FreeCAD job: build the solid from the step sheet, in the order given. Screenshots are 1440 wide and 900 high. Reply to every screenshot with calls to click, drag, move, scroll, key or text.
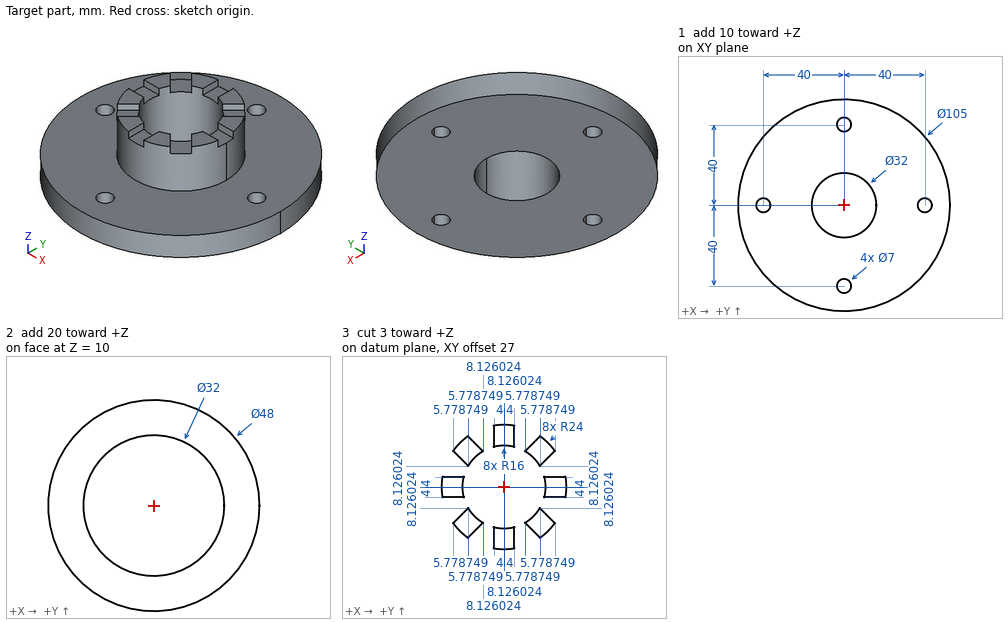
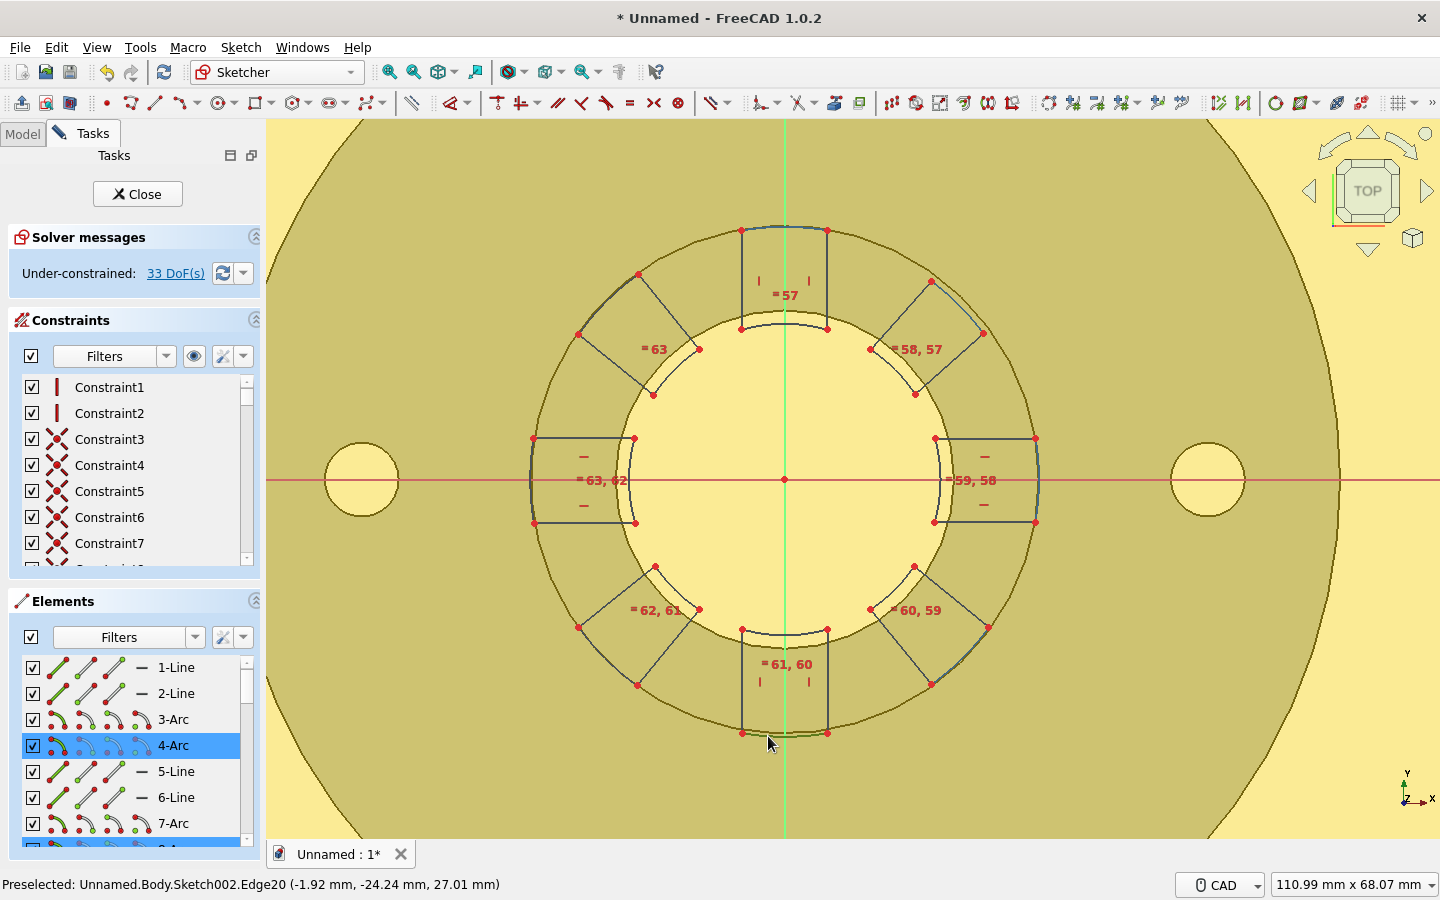
click(594, 647)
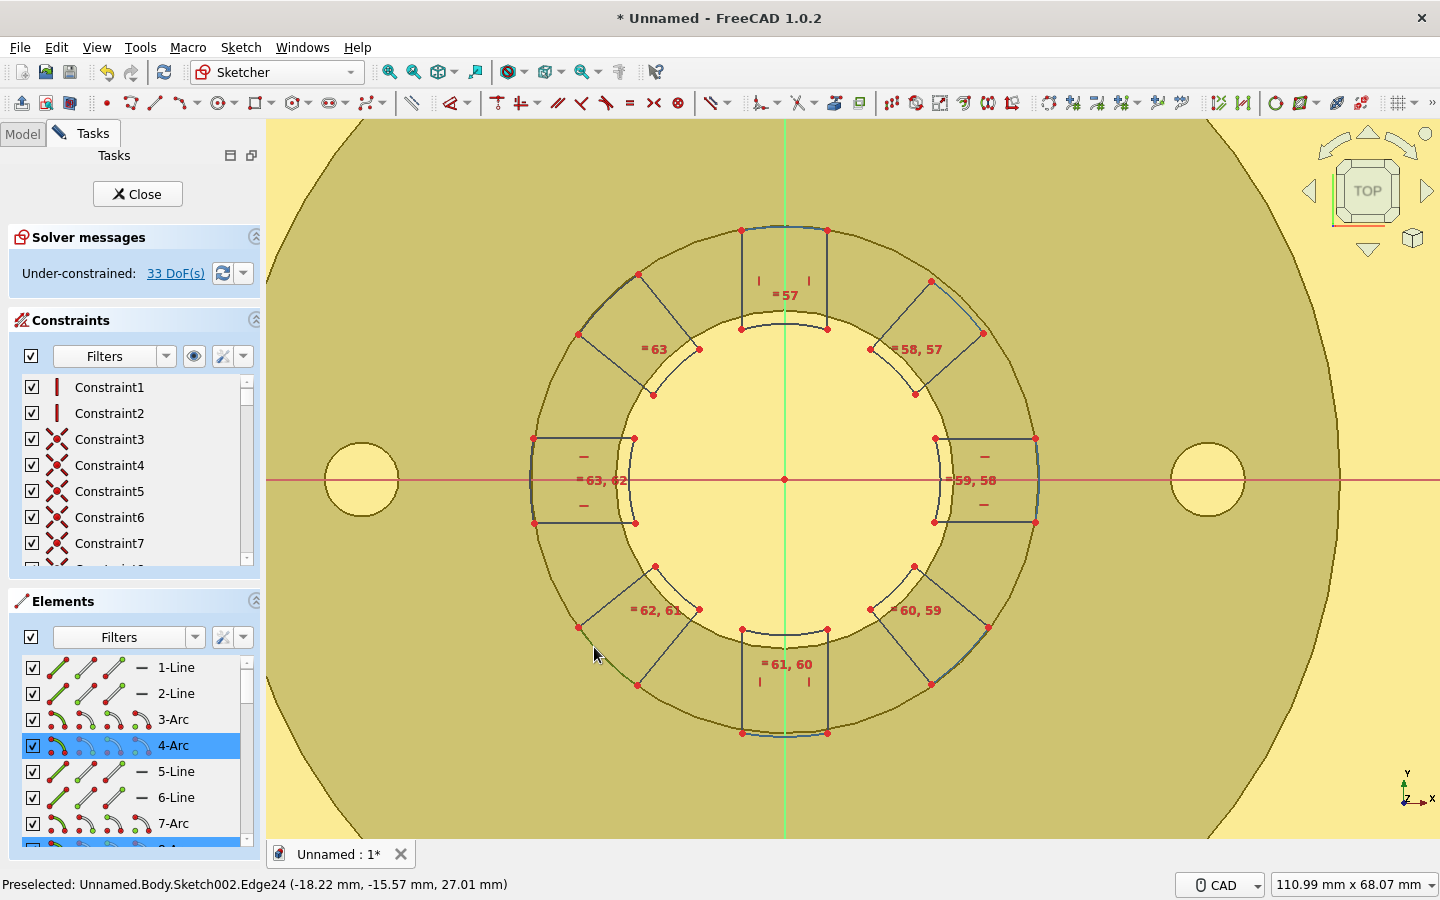
click(531, 464)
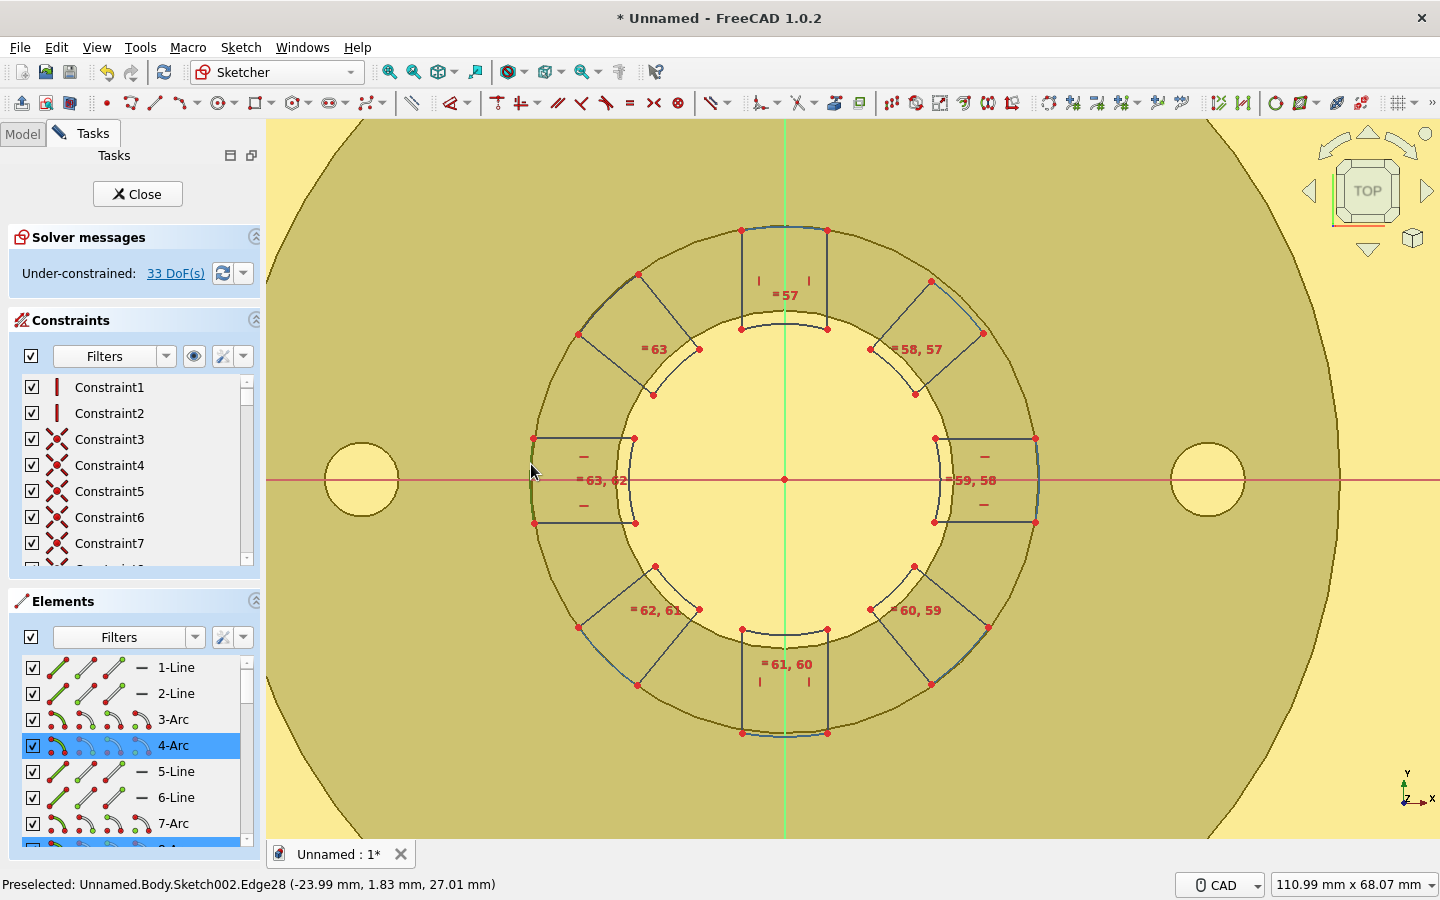
click(618, 290)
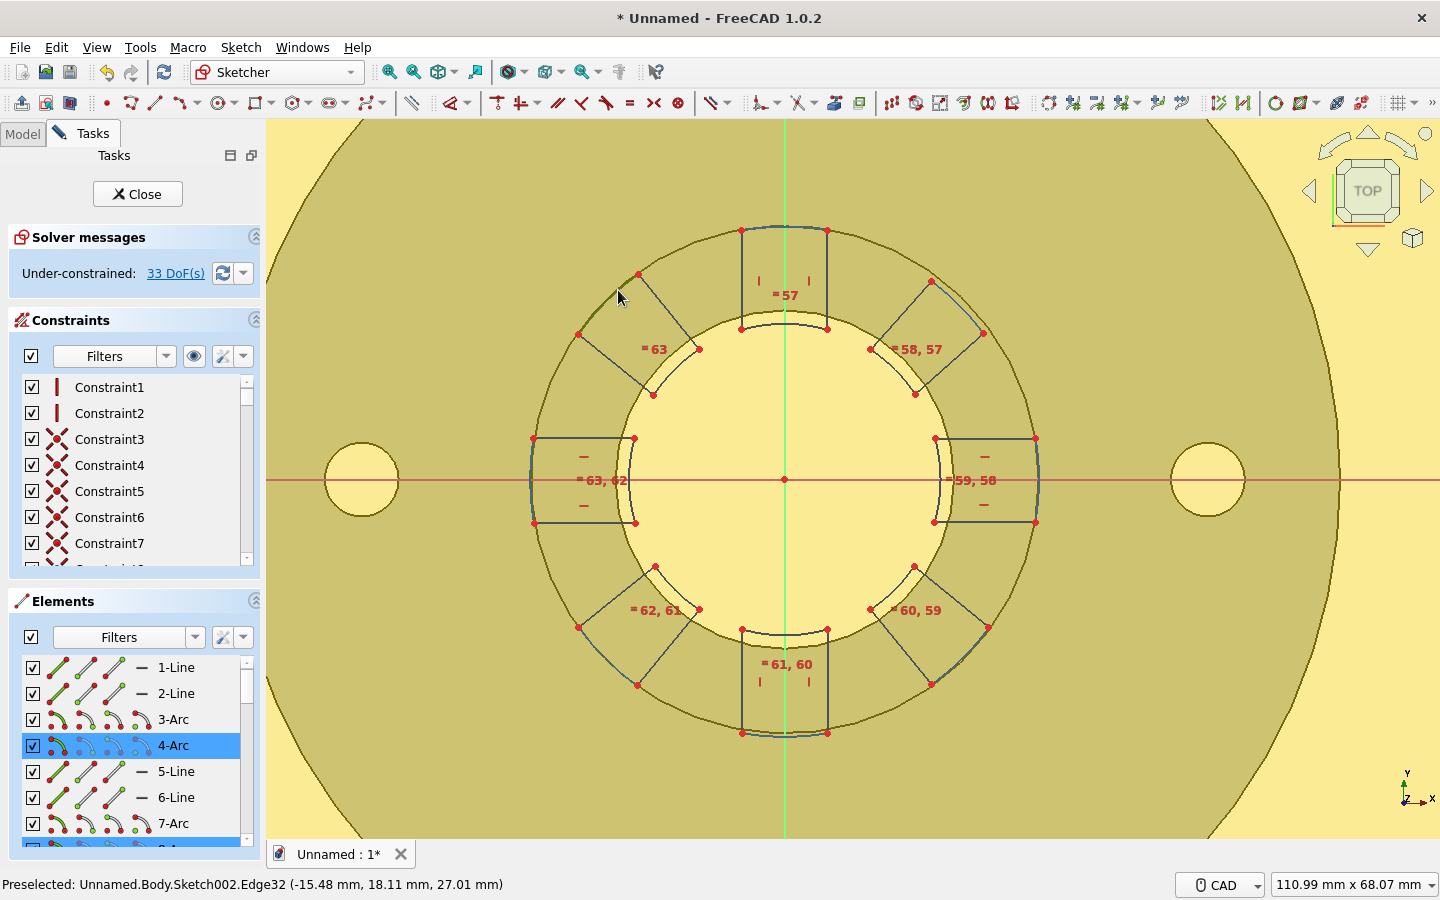
click(630, 104)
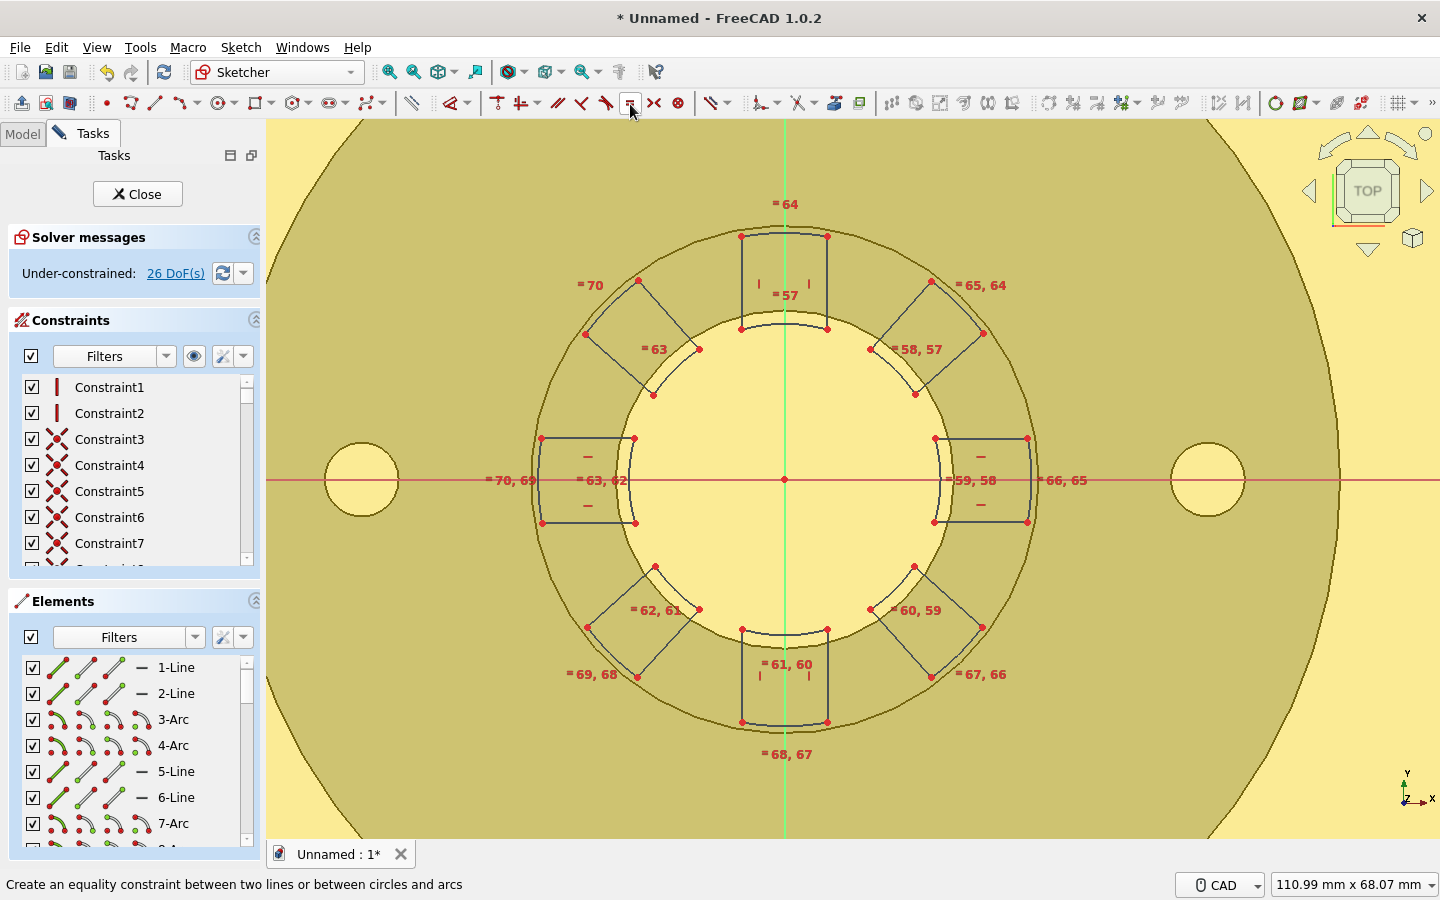
click(450, 104)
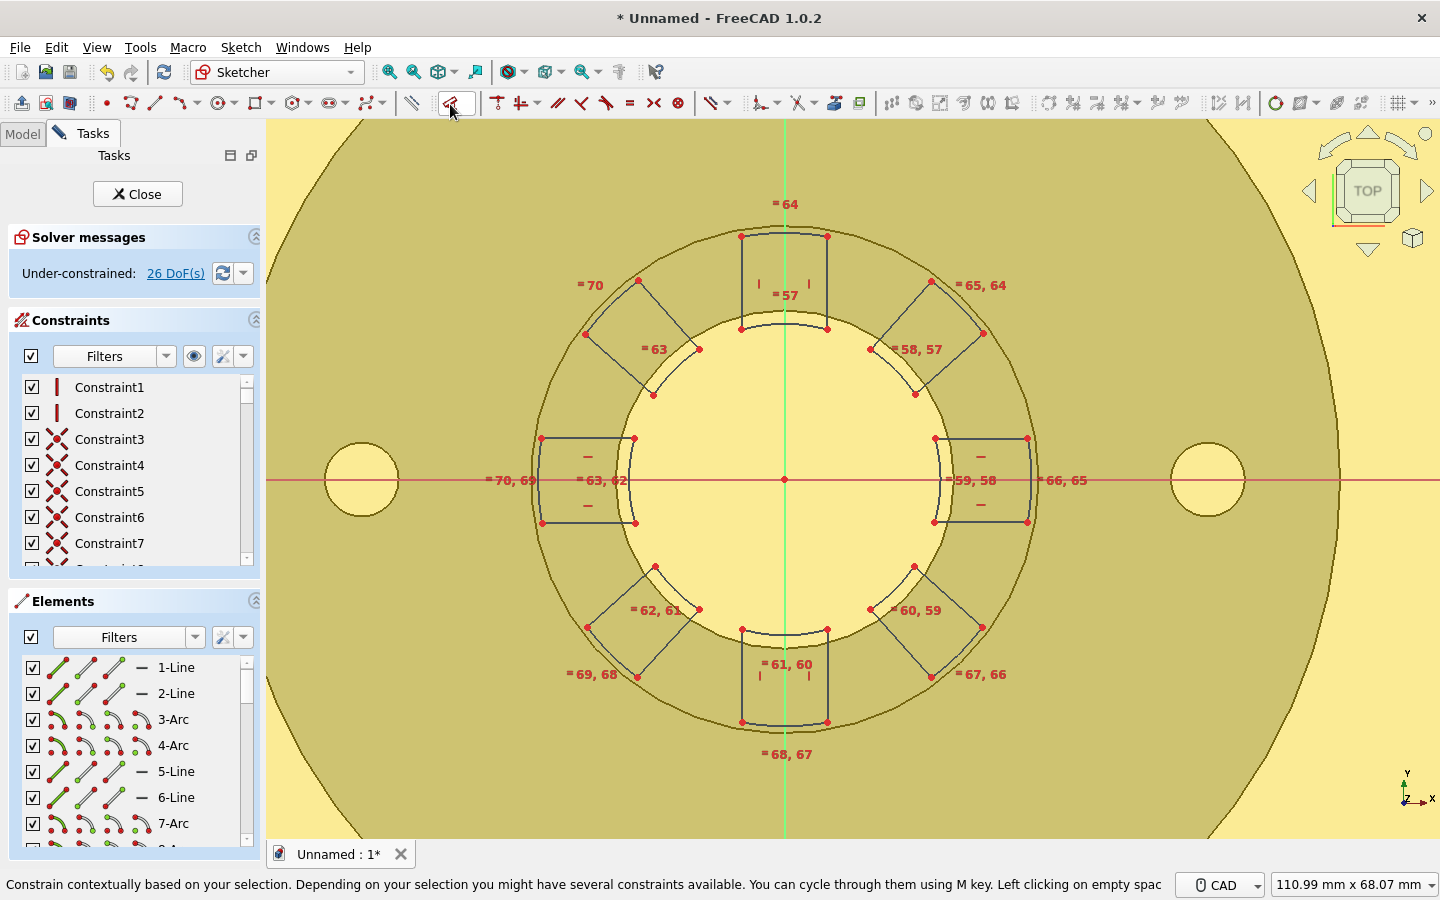
click(802, 325)
click(806, 293)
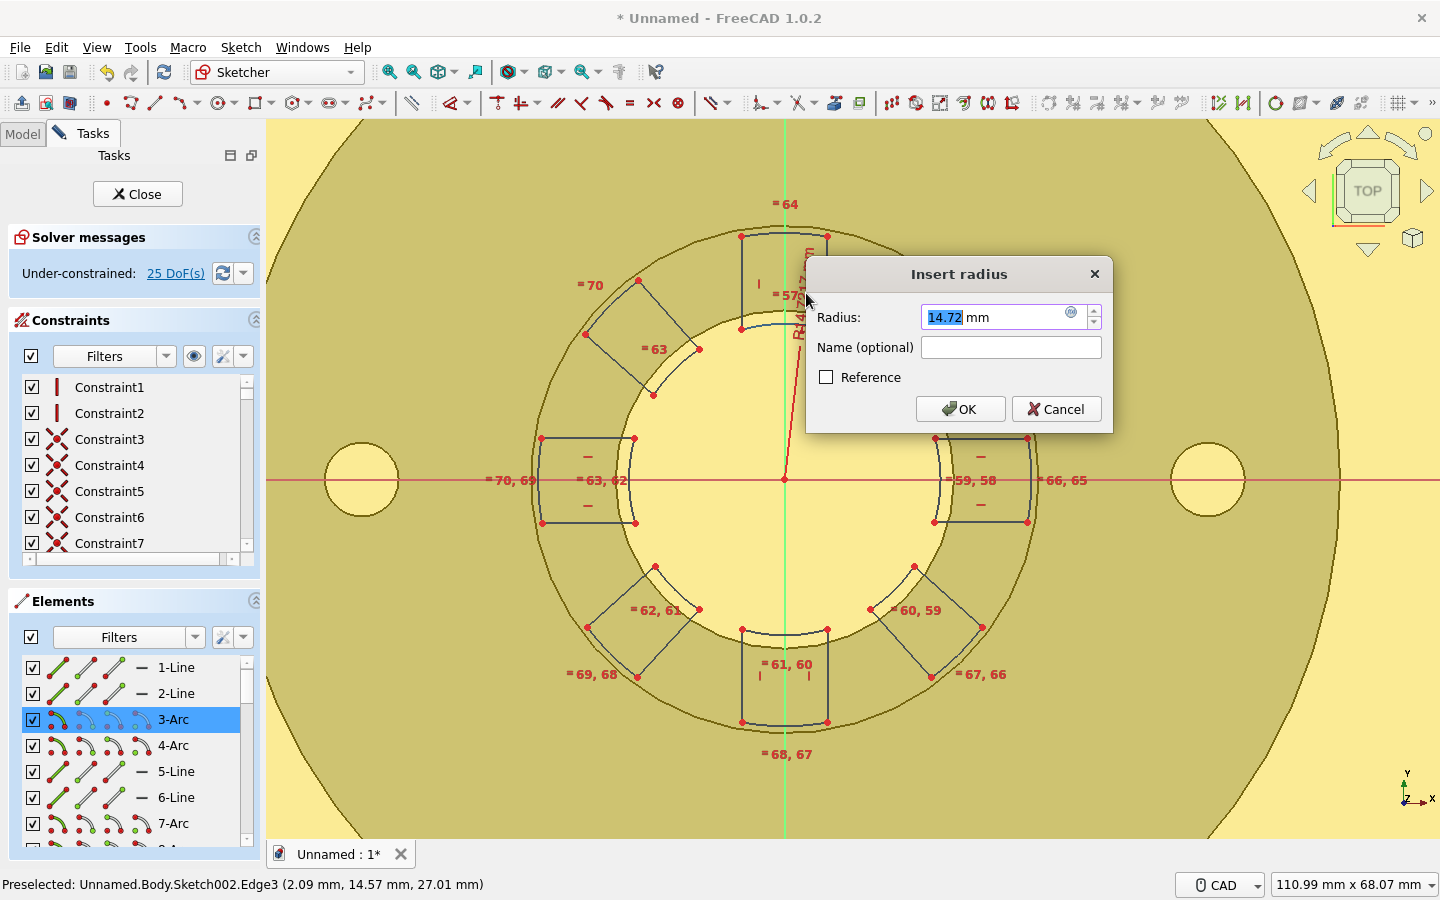
text(16)
key(Return)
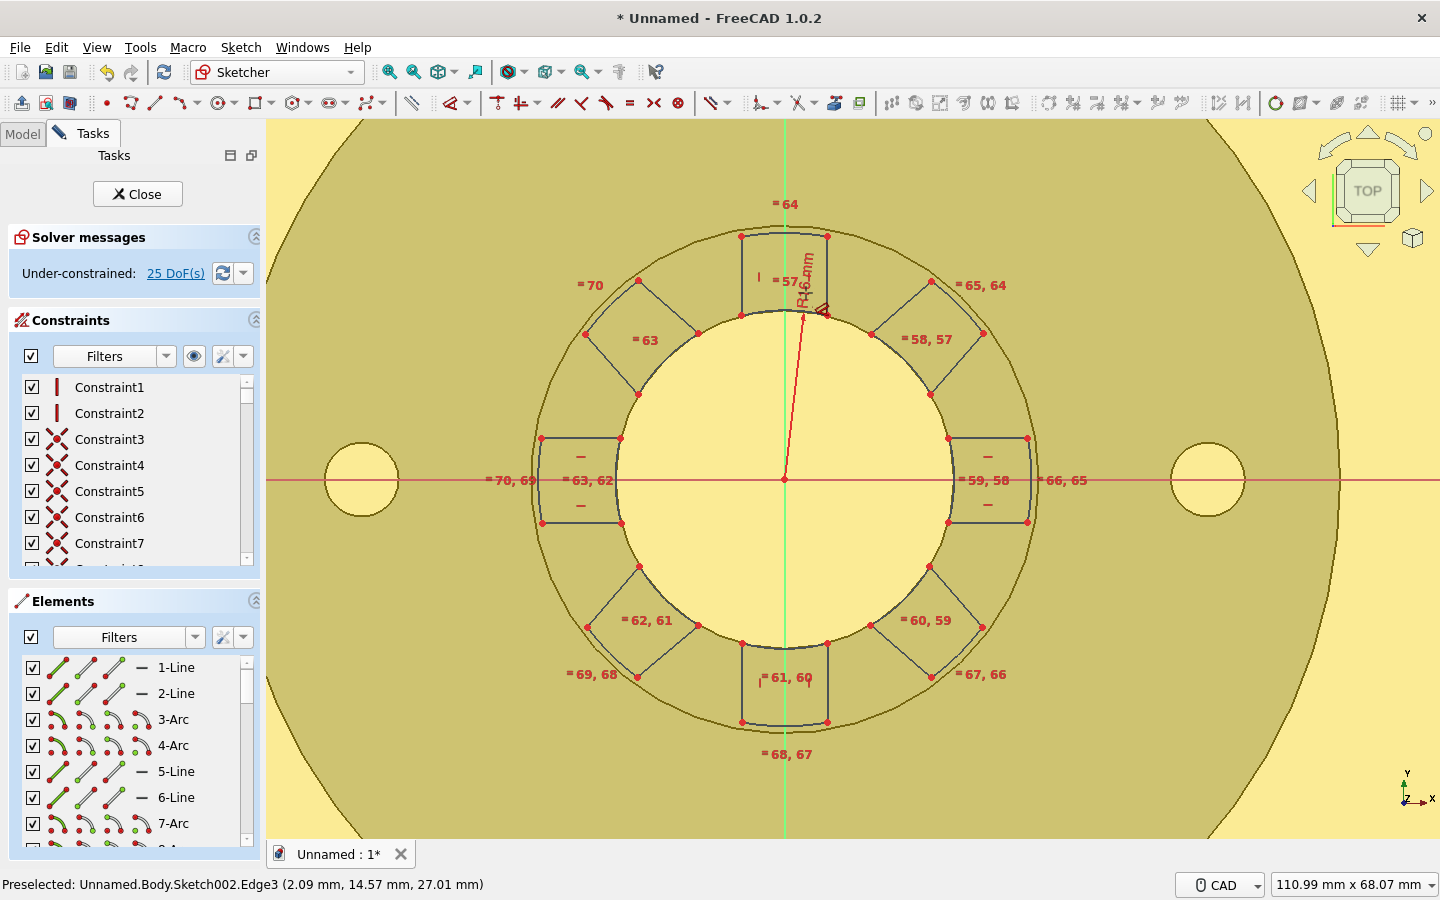
click(802, 234)
click(804, 202)